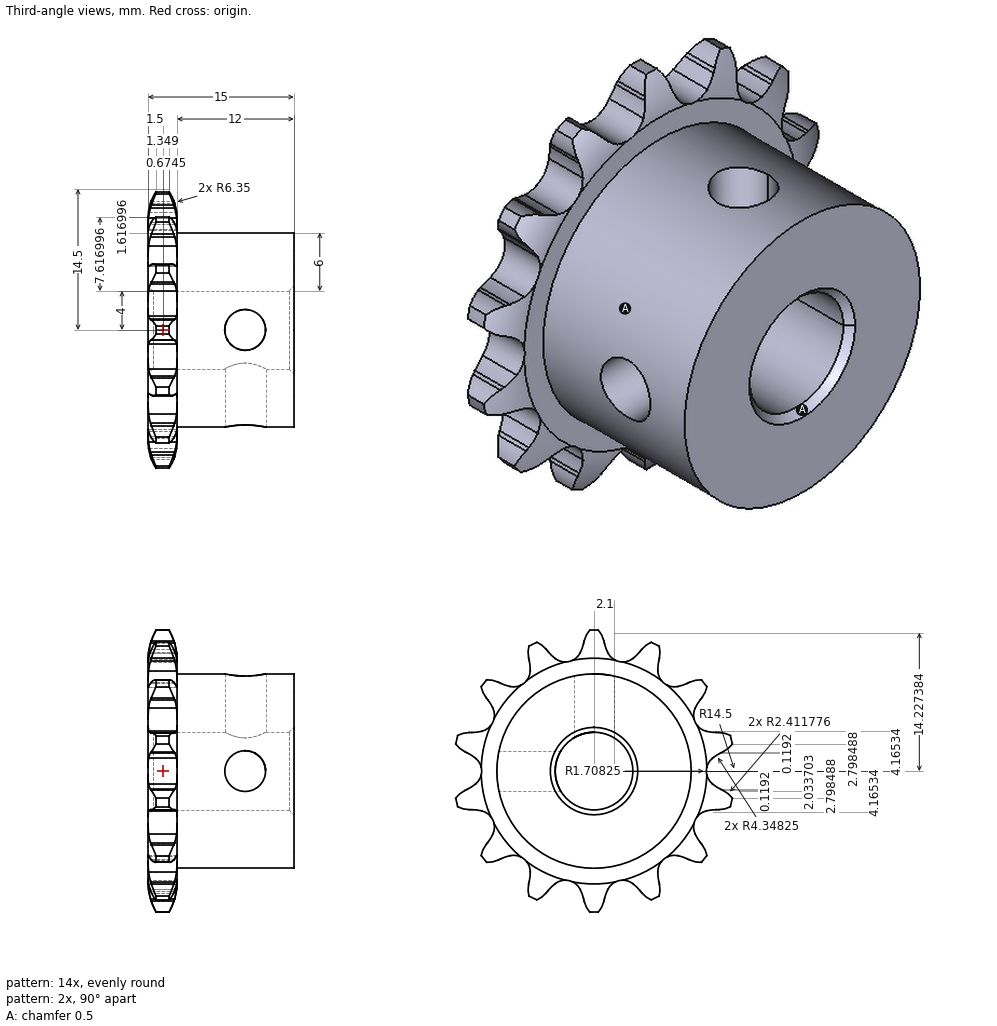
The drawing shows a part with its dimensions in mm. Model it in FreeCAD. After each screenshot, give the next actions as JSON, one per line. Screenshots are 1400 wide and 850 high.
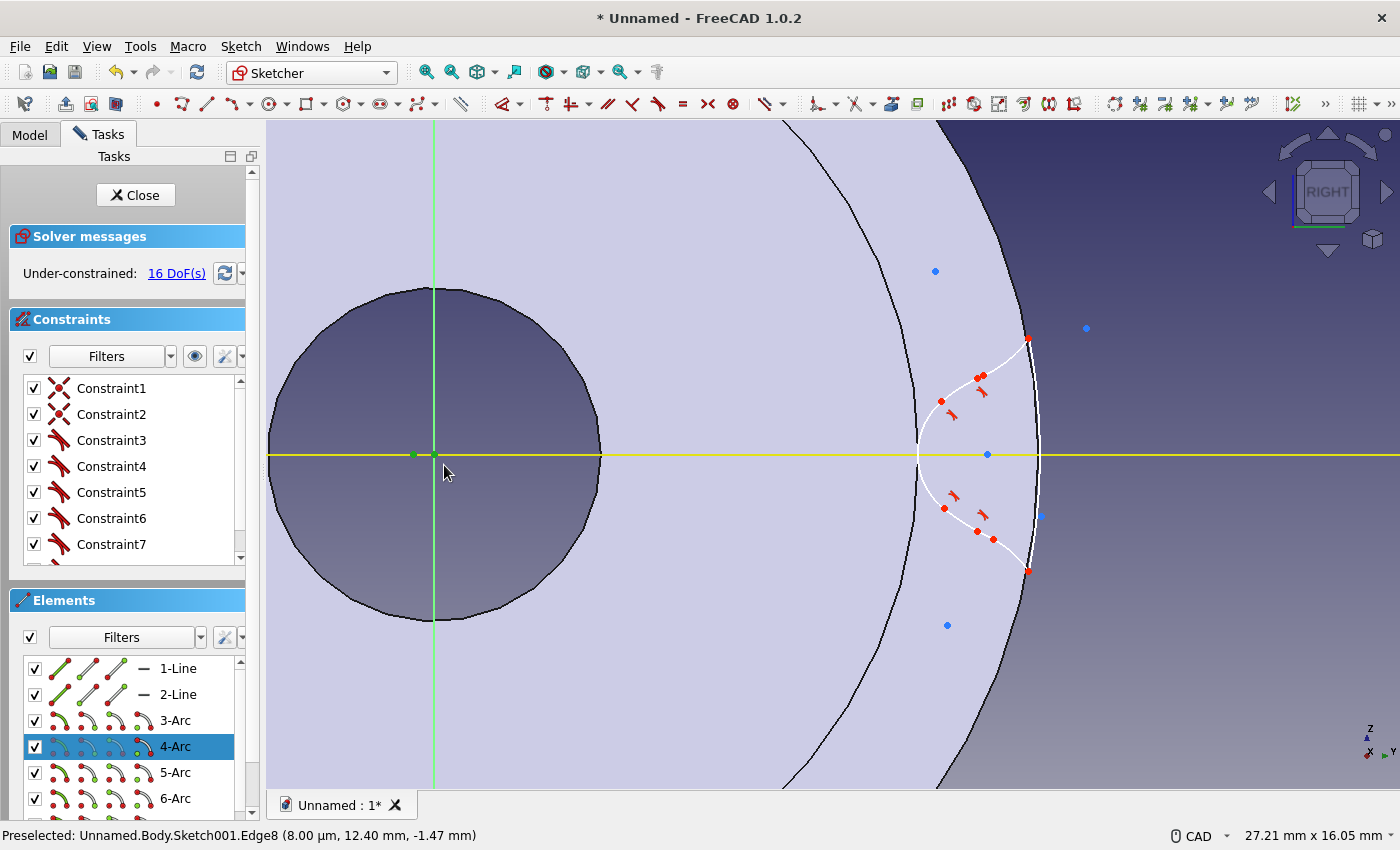
{"action": "left_click", "coordinate": [546, 104]}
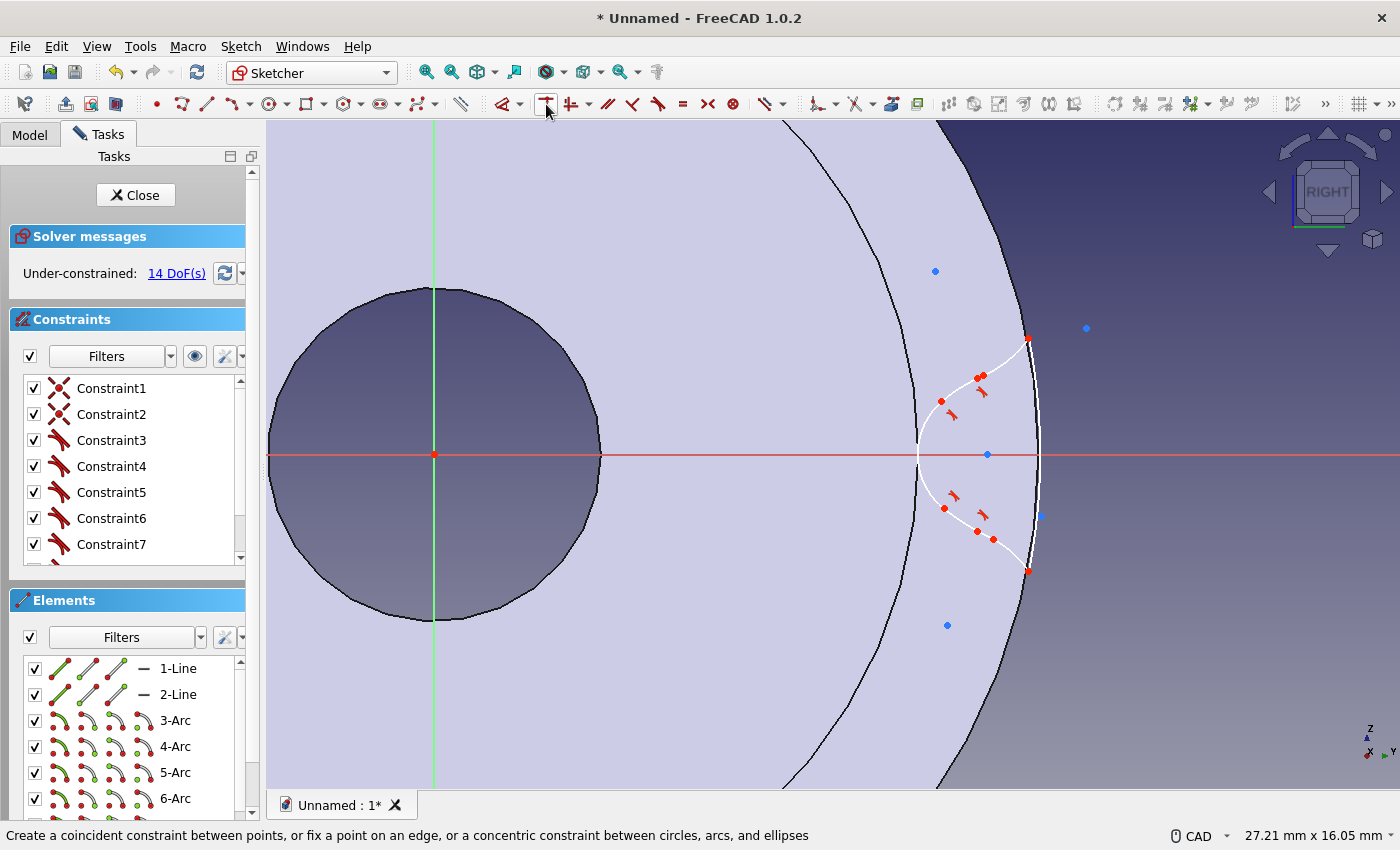
{"action": "scroll", "coordinate": [1020, 560], "scroll_direction": "up", "scroll_amount": 2}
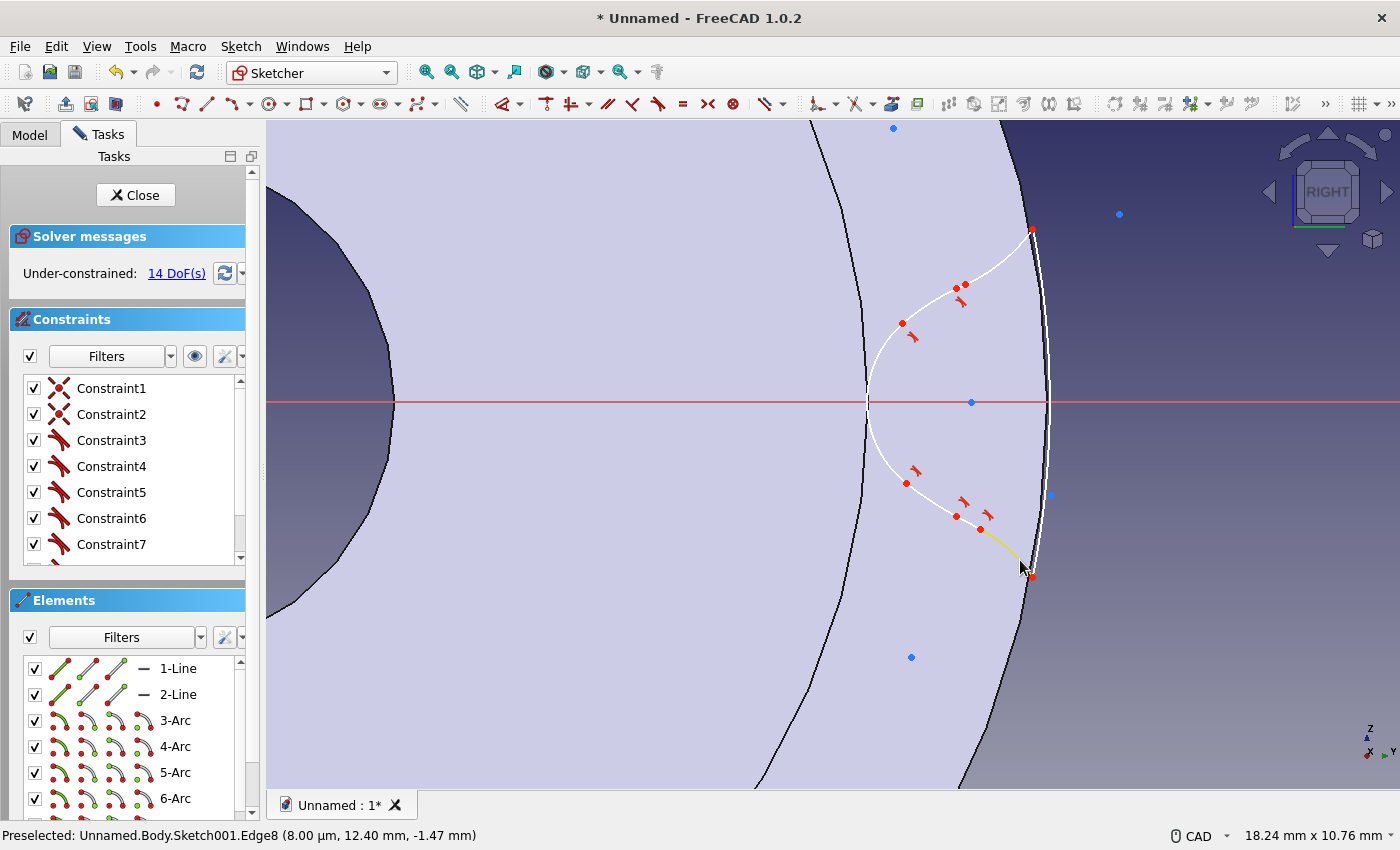
{"action": "left_click", "coordinate": [1020, 560]}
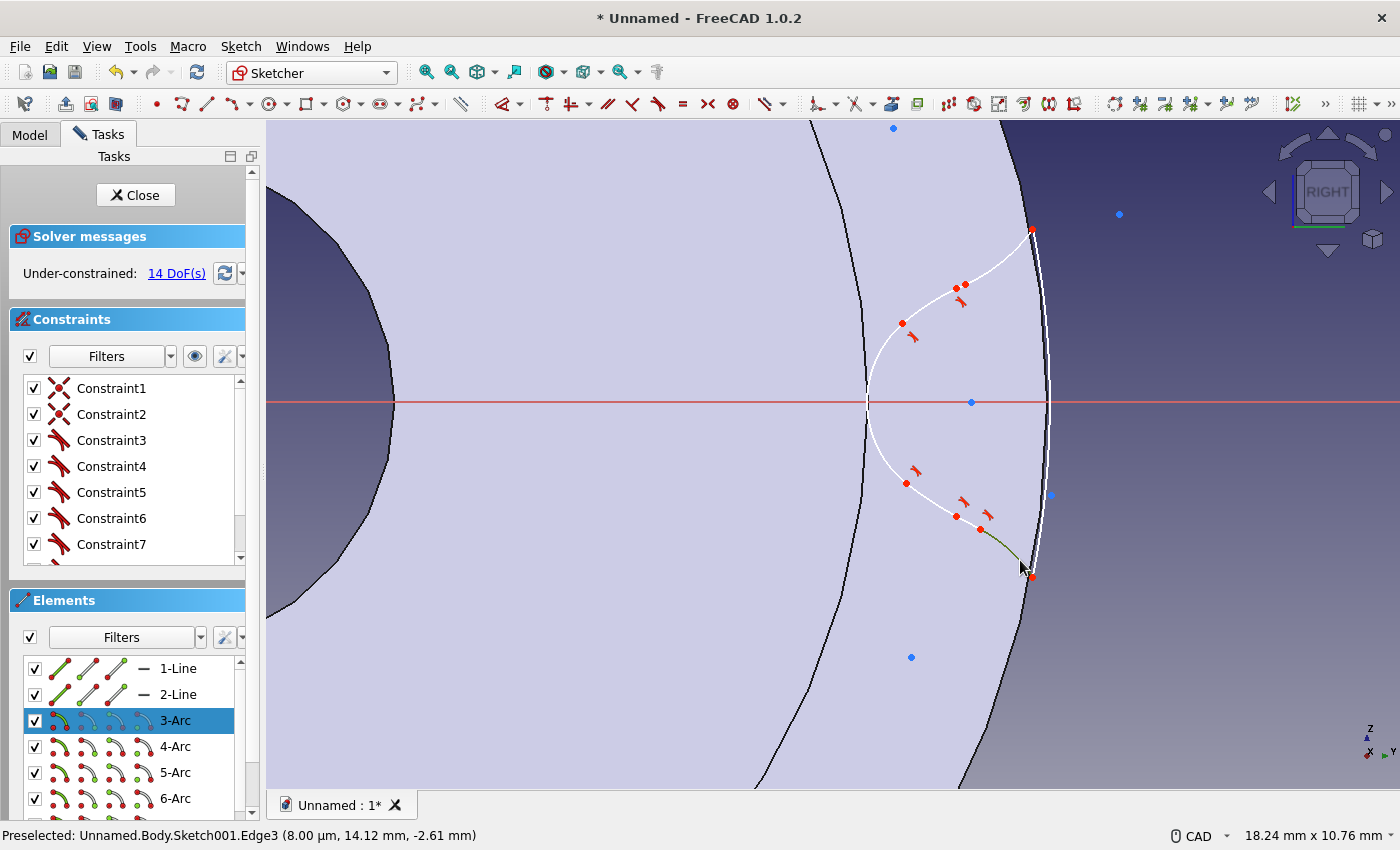
{"action": "left_click", "coordinate": [989, 272]}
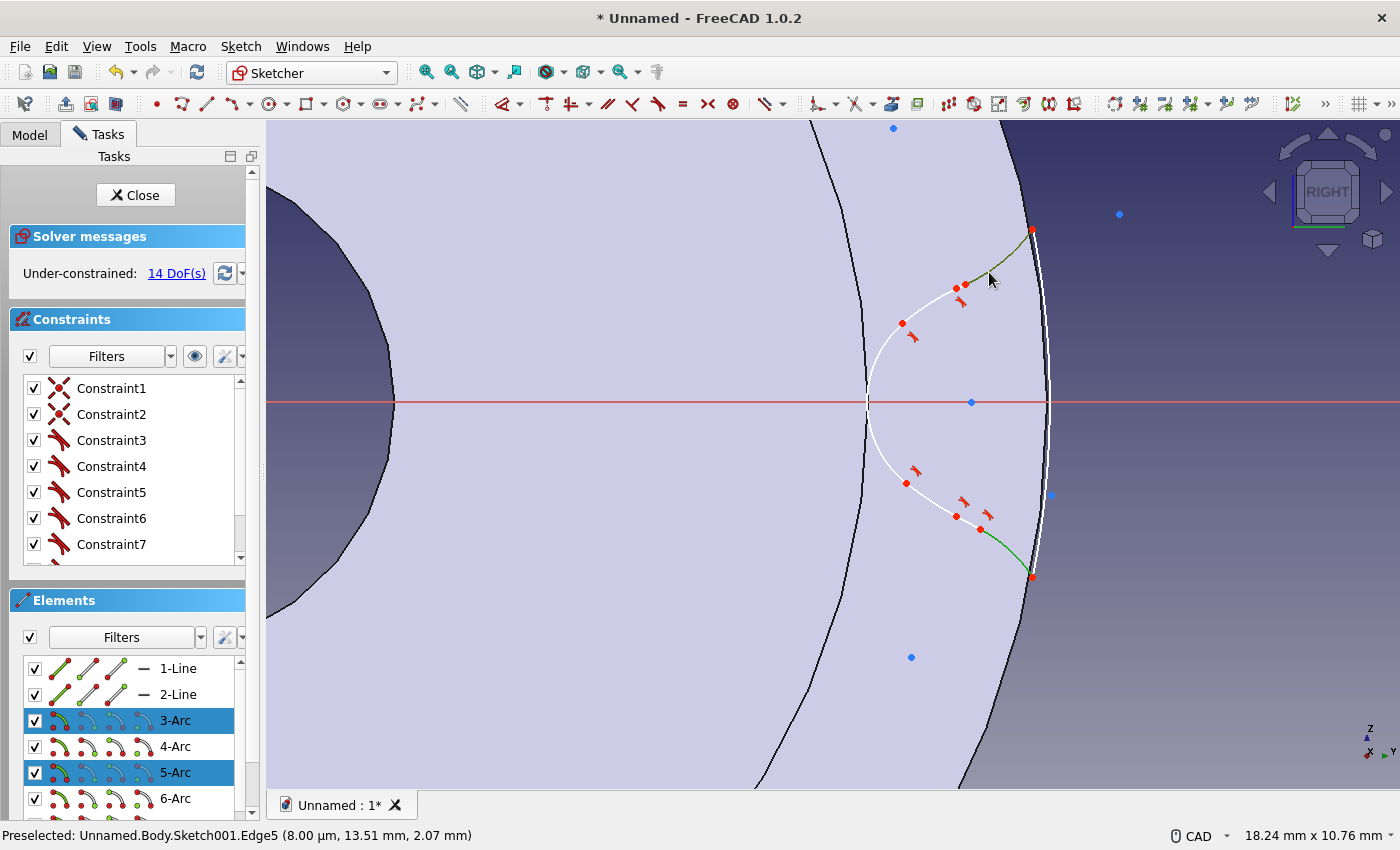
{"action": "key", "text": "e"}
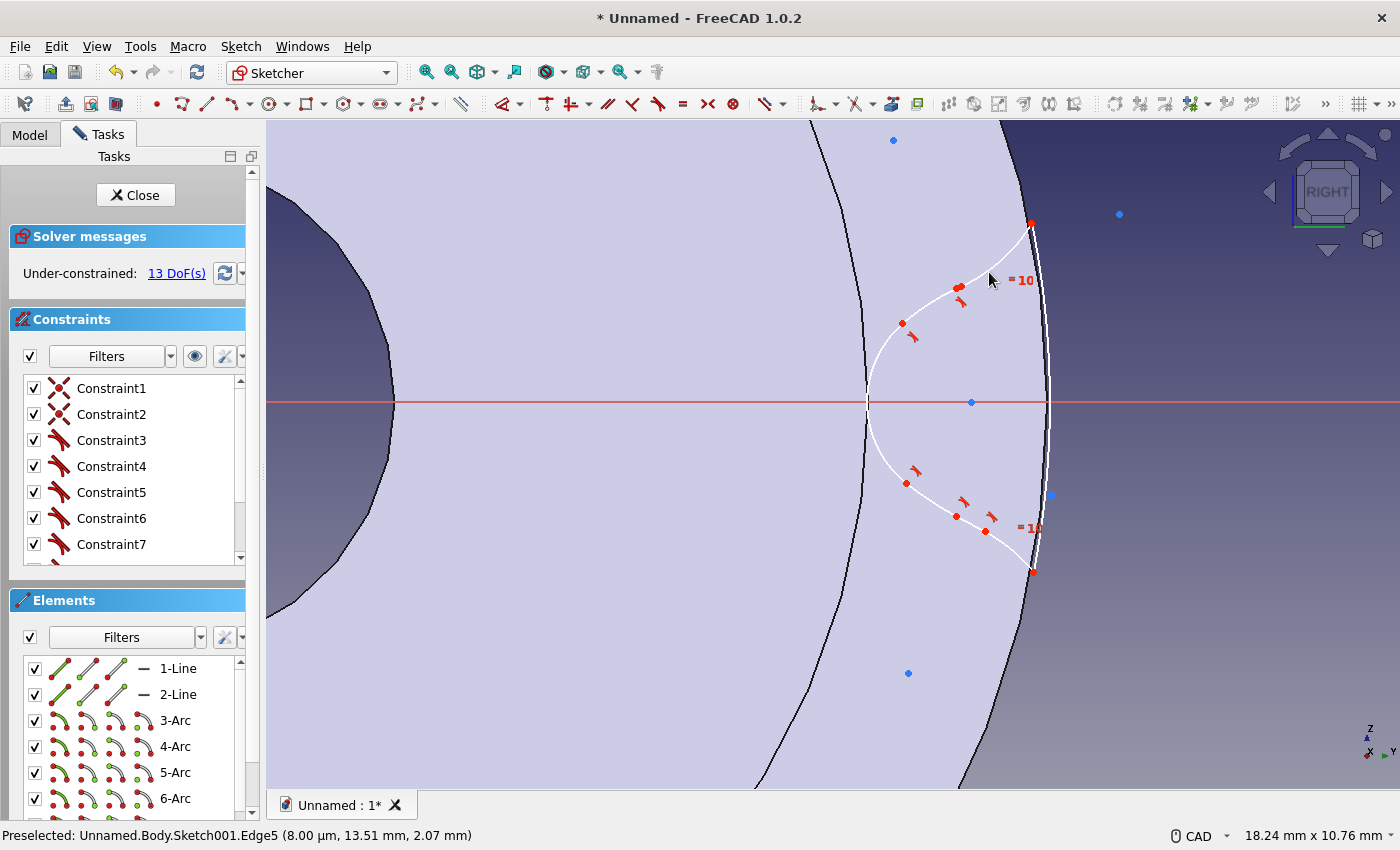
{"action": "left_click", "coordinate": [940, 298]}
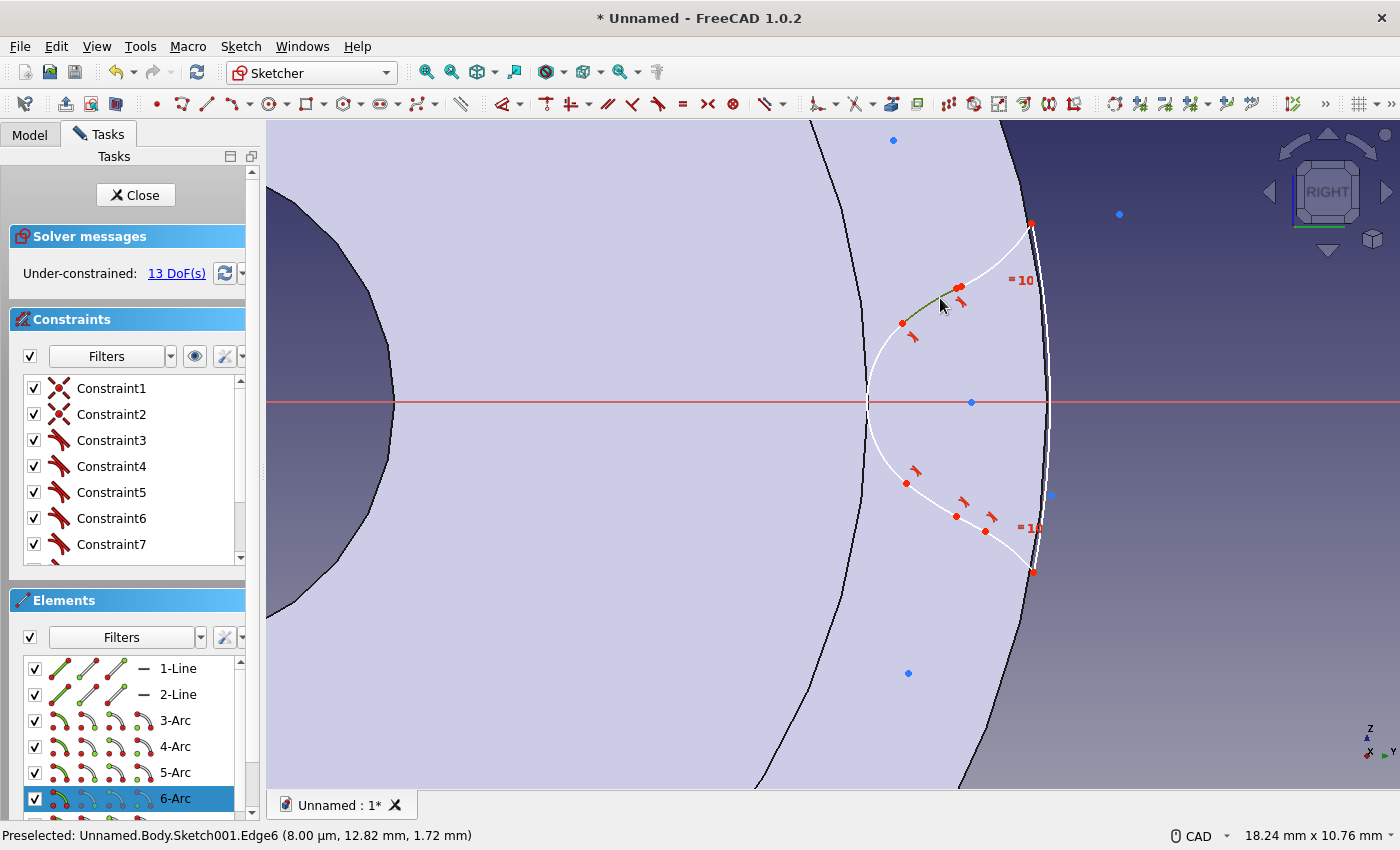
{"action": "left_click", "coordinate": [921, 494]}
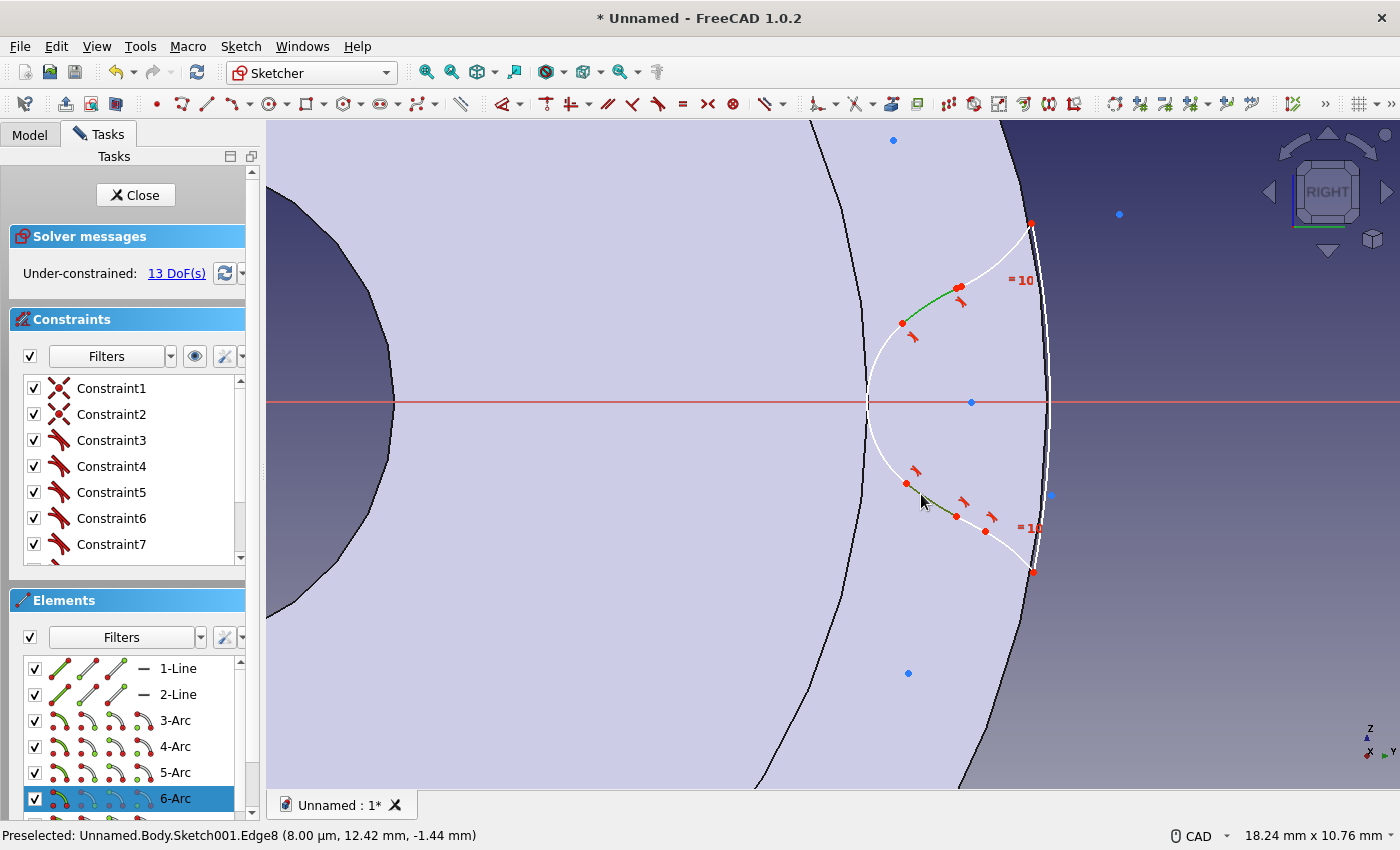
{"action": "left_click", "coordinate": [683, 104]}